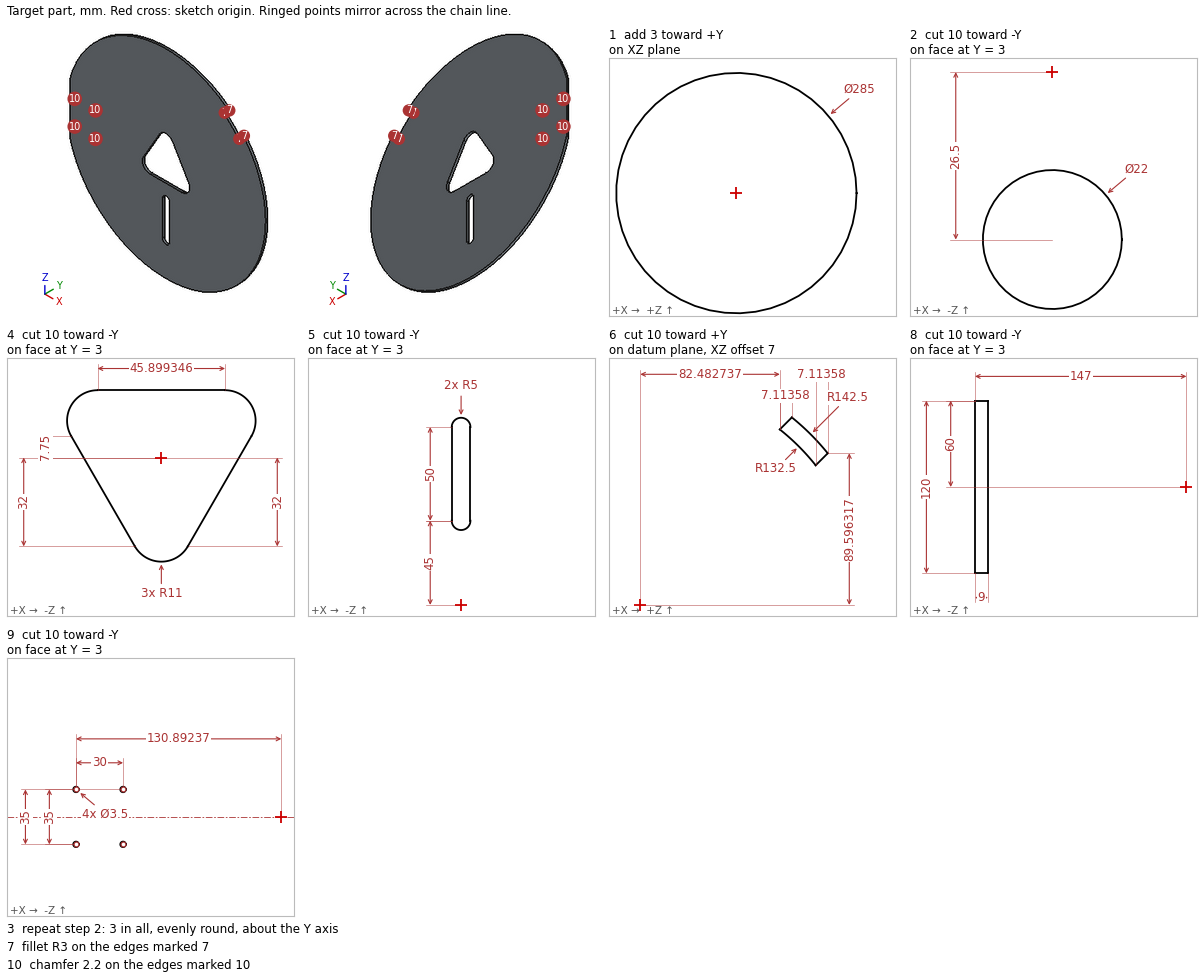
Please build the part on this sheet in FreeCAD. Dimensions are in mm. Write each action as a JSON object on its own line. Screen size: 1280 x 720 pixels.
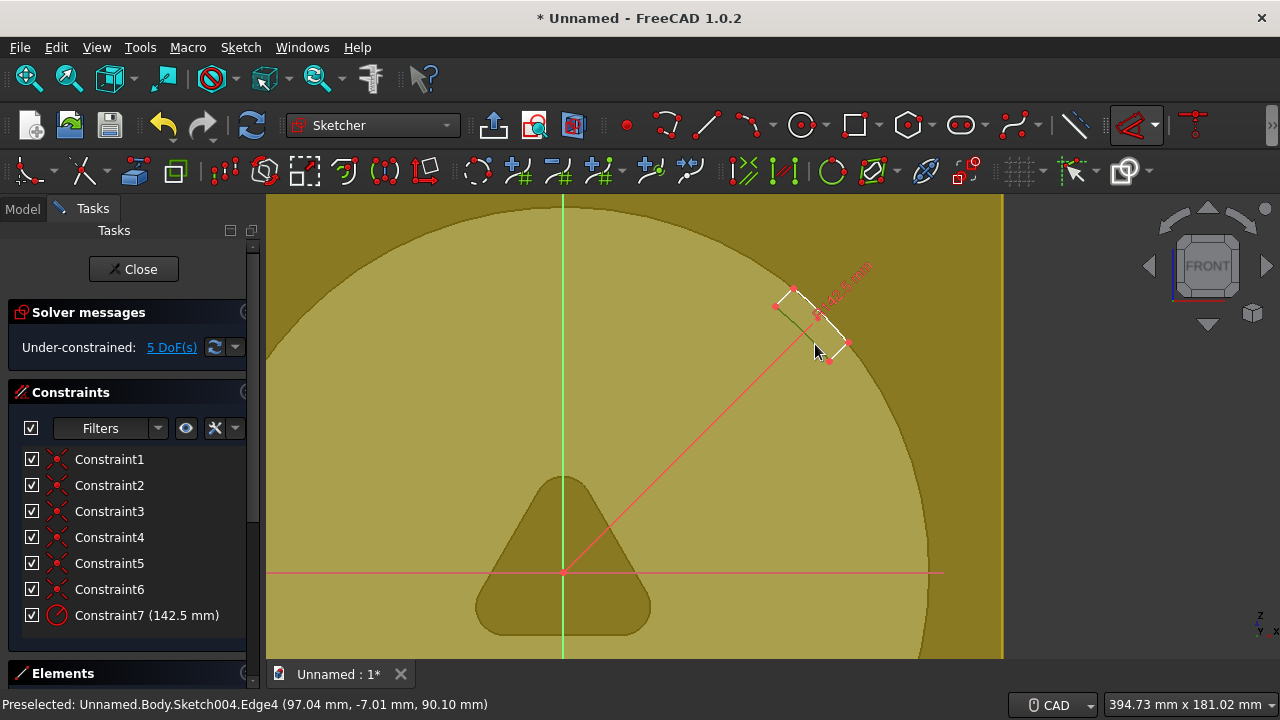
{"action": "left_click", "coordinate": [1158, 126]}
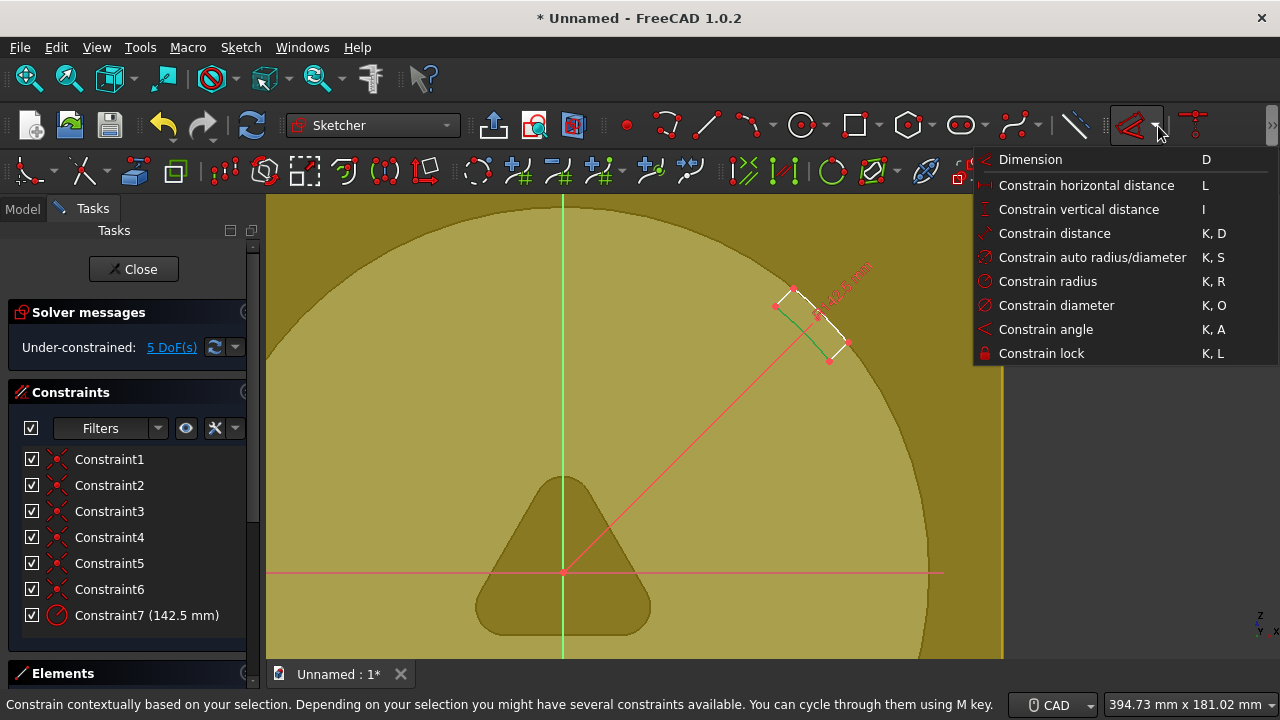
{"action": "left_click", "coordinate": [1126, 281]}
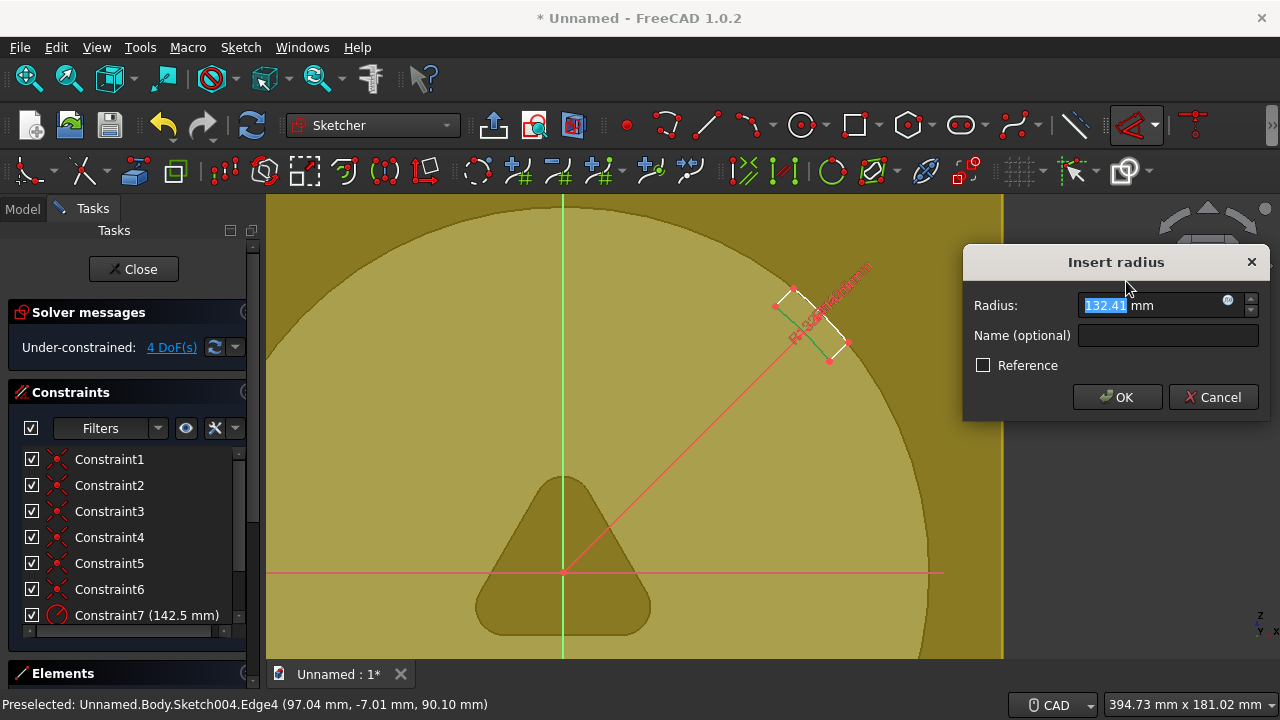
{"action": "type", "text": "132.5"}
{"action": "key", "text": "Return"}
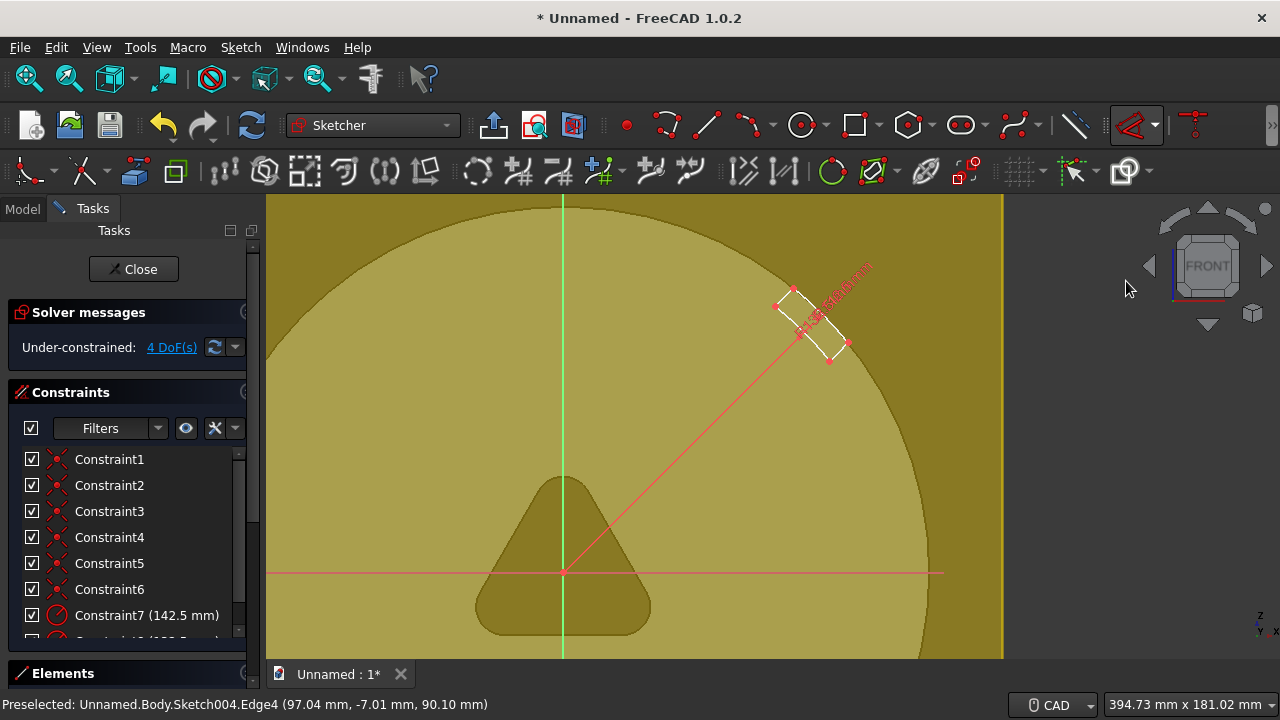
{"action": "scroll", "coordinate": [783, 299], "scroll_direction": "up", "scroll_amount": 4}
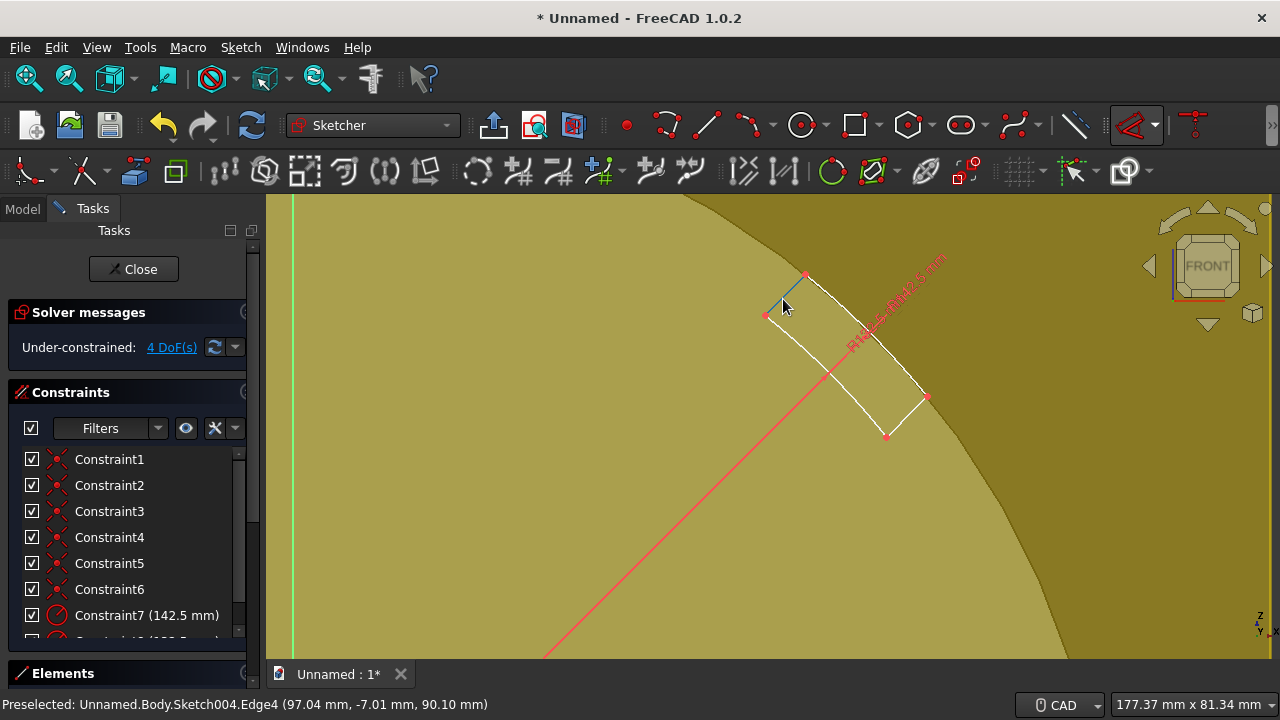
{"action": "left_click", "coordinate": [781, 299]}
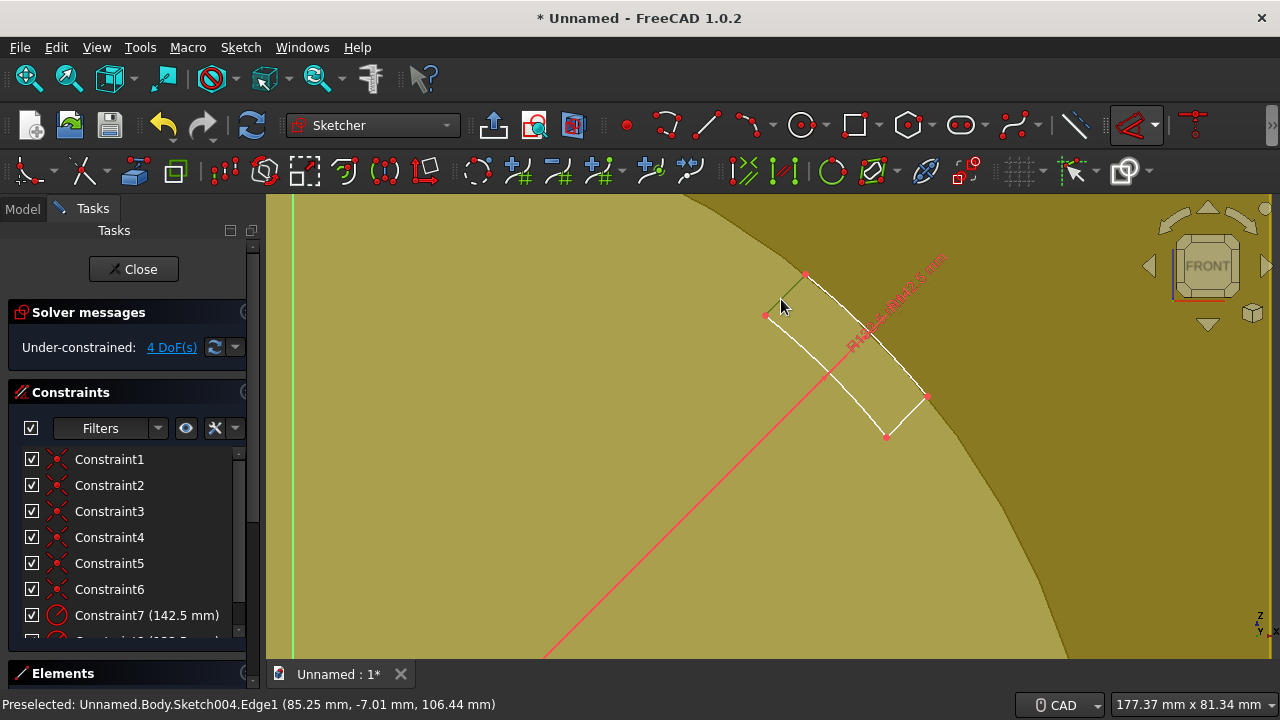
{"action": "left_click", "coordinate": [1158, 126]}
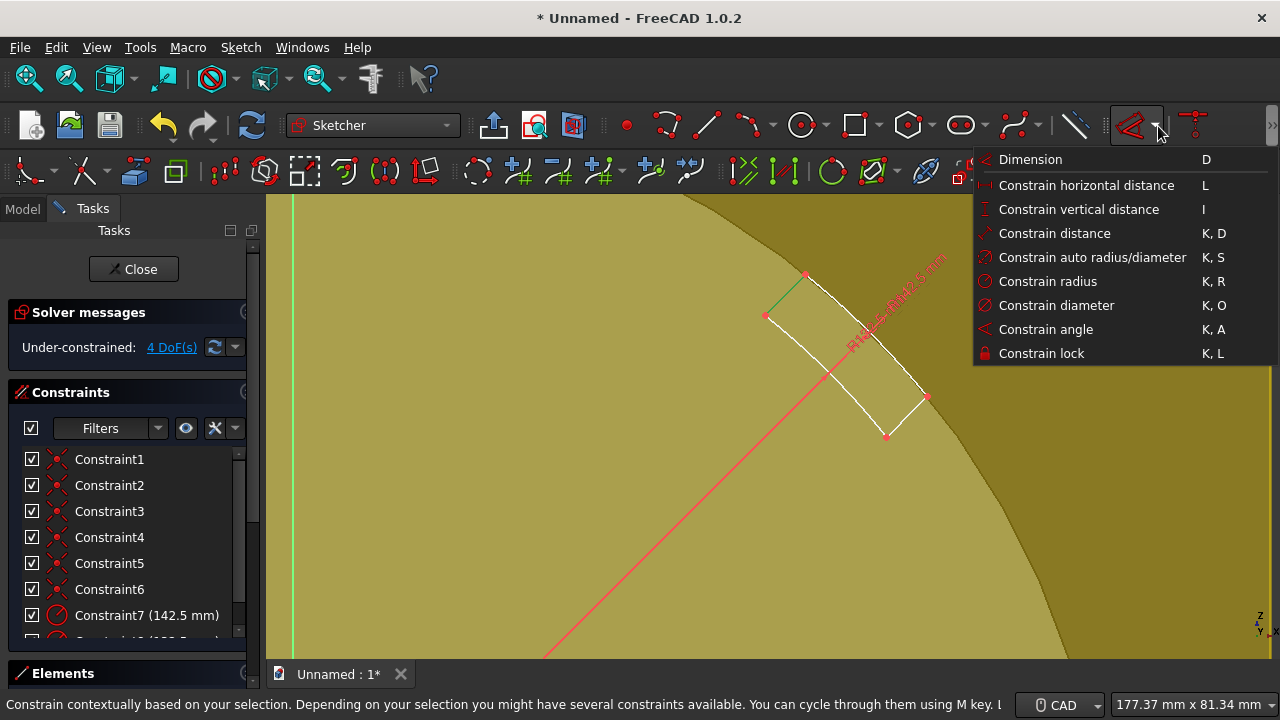
{"action": "left_click", "coordinate": [1126, 185]}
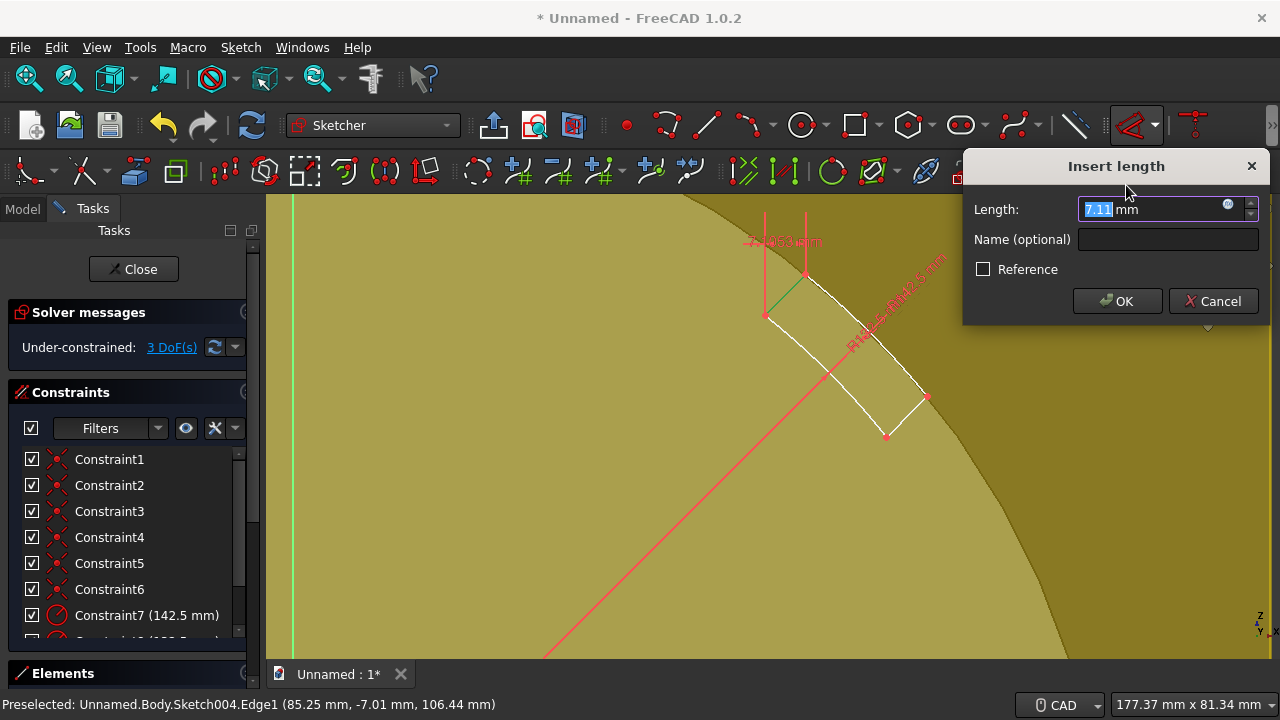
{"action": "type", "text": "7.11358"}
{"action": "key", "text": "Return"}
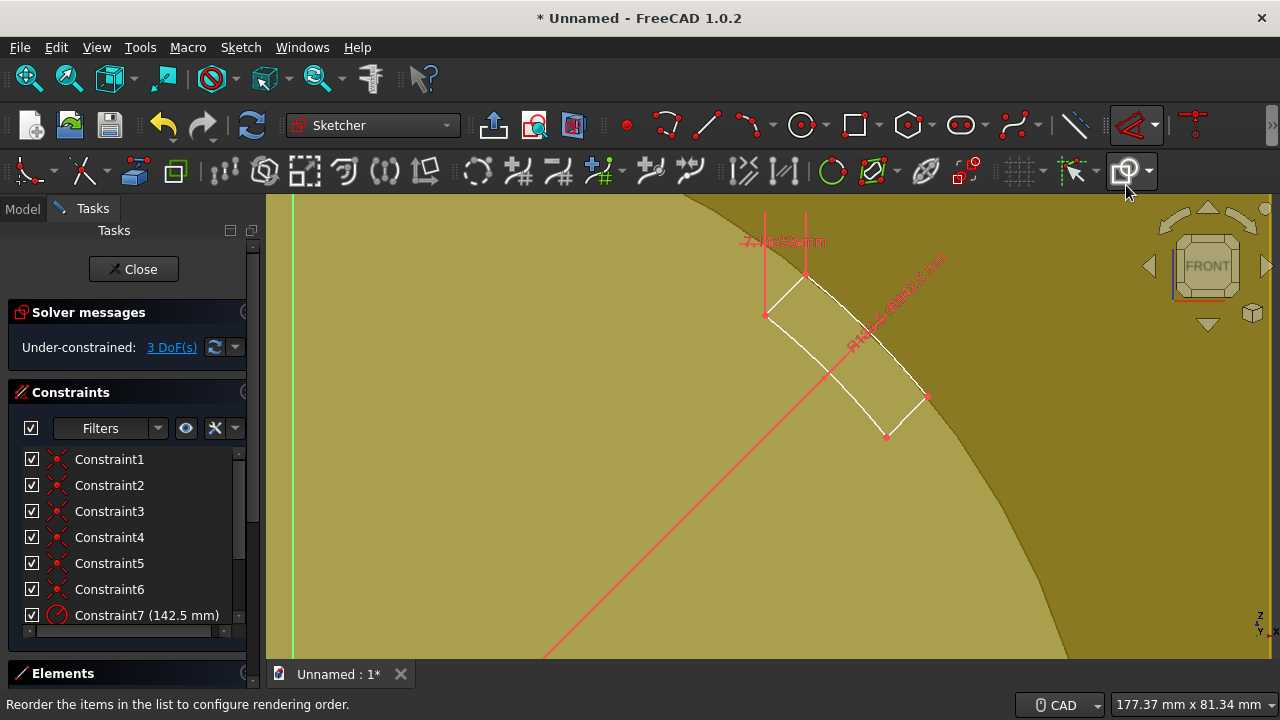
{"action": "left_click", "coordinate": [915, 409]}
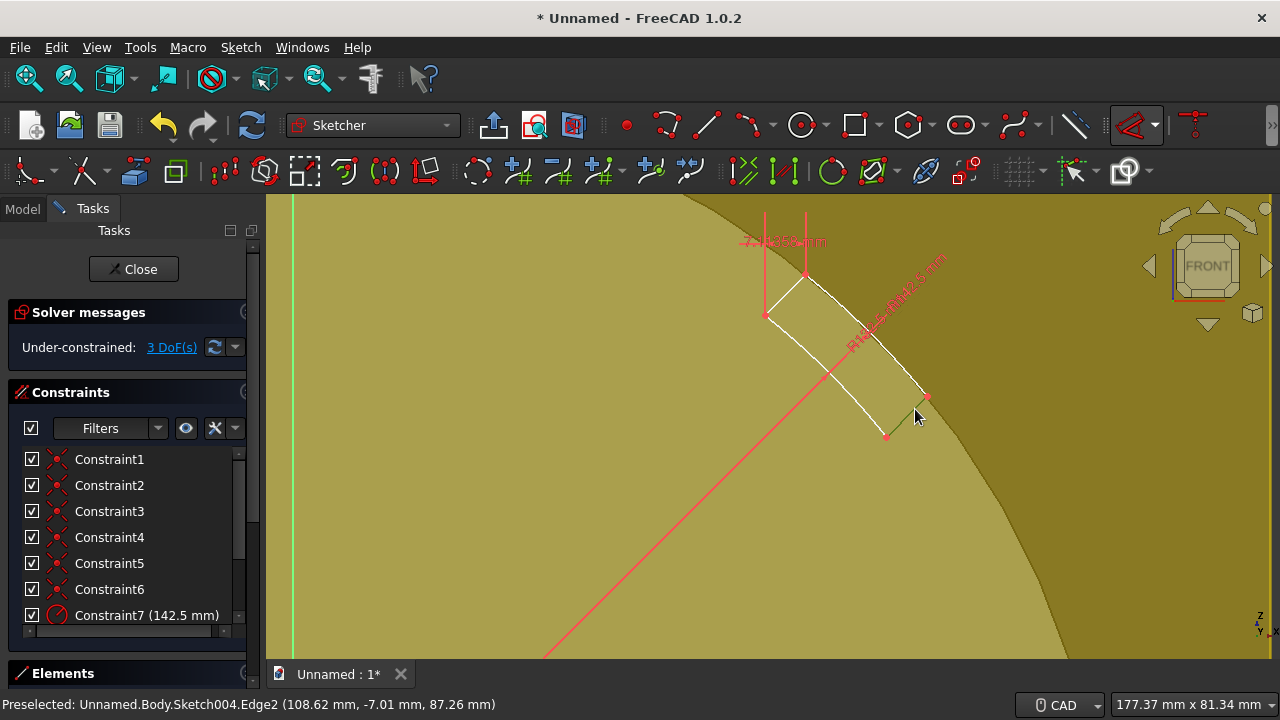
{"action": "key", "text": "l"}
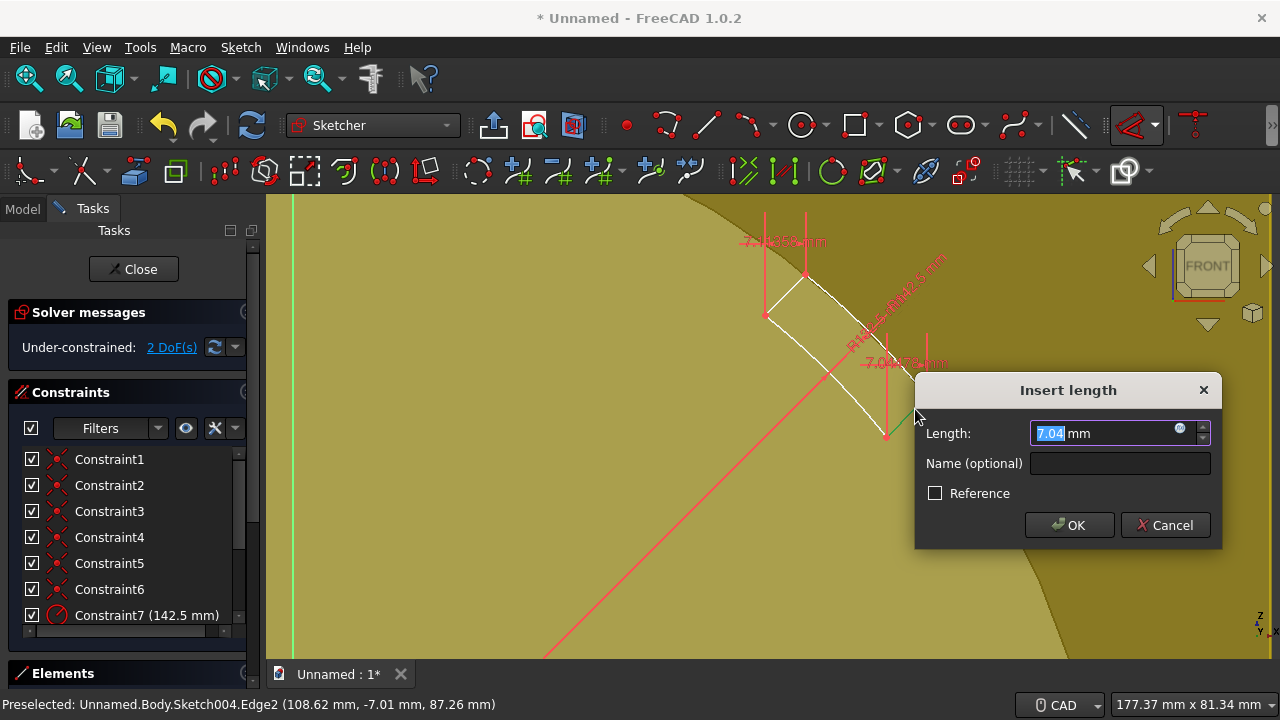
{"action": "type", "text": "7.11358"}
{"action": "key", "text": "Return"}